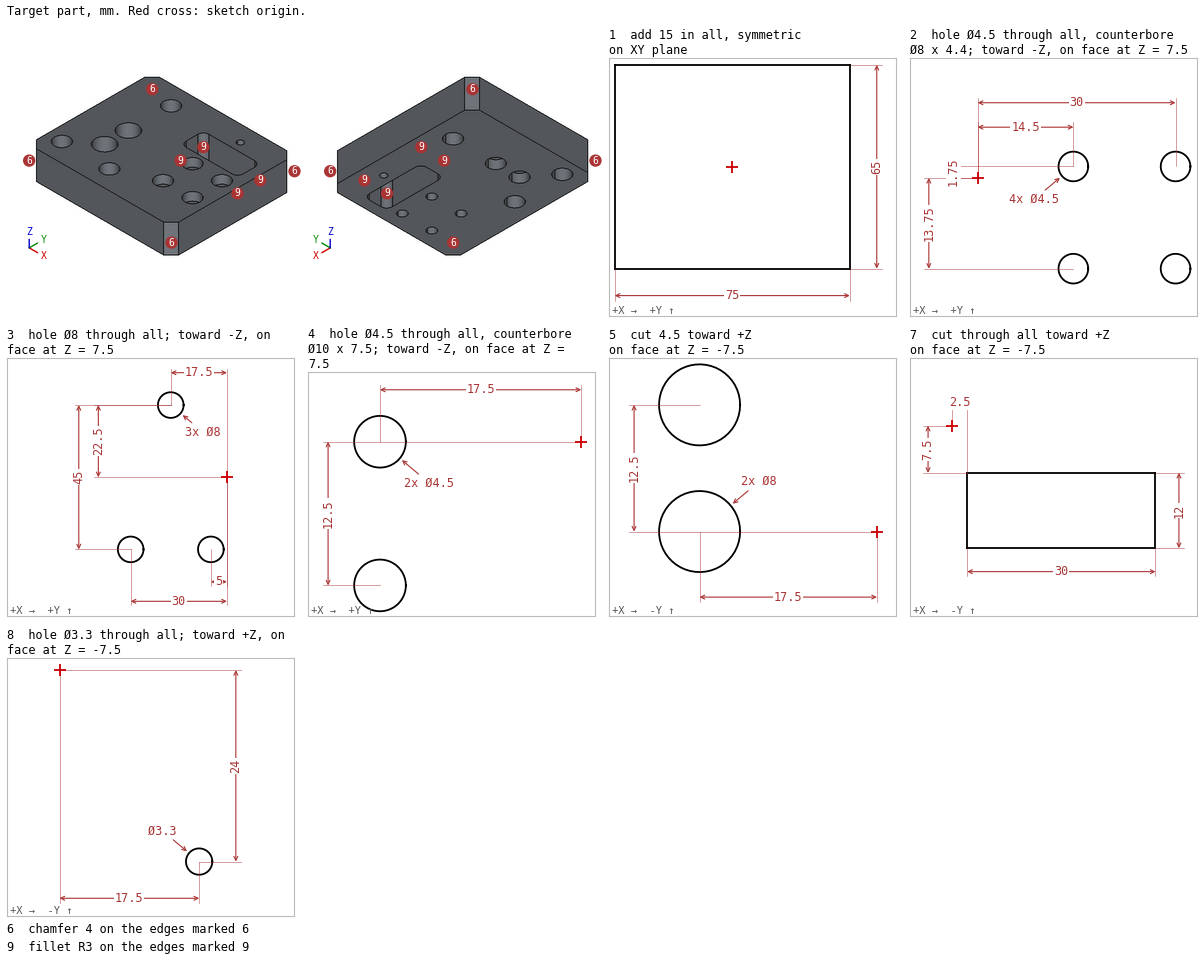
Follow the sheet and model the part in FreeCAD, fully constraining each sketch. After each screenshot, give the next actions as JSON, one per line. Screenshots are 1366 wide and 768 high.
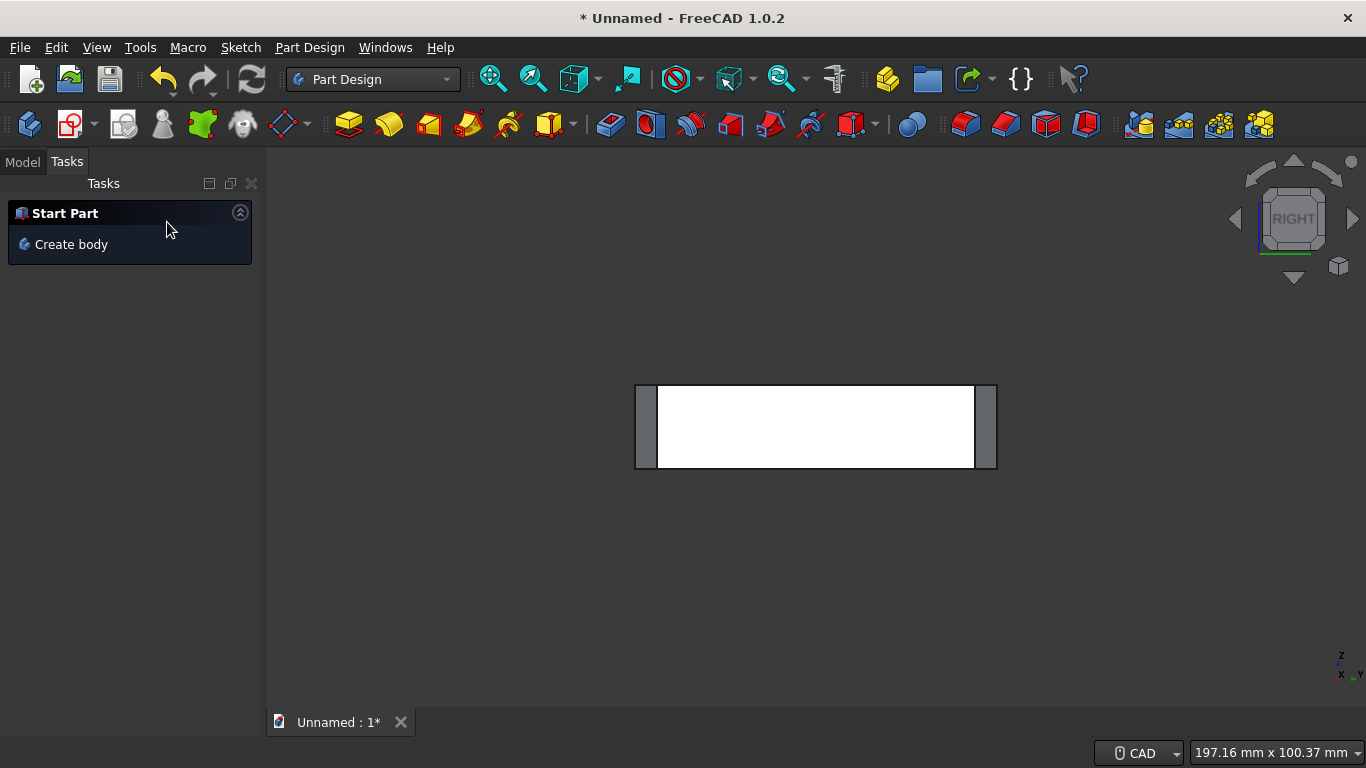
{"action": "key", "text": "v f"}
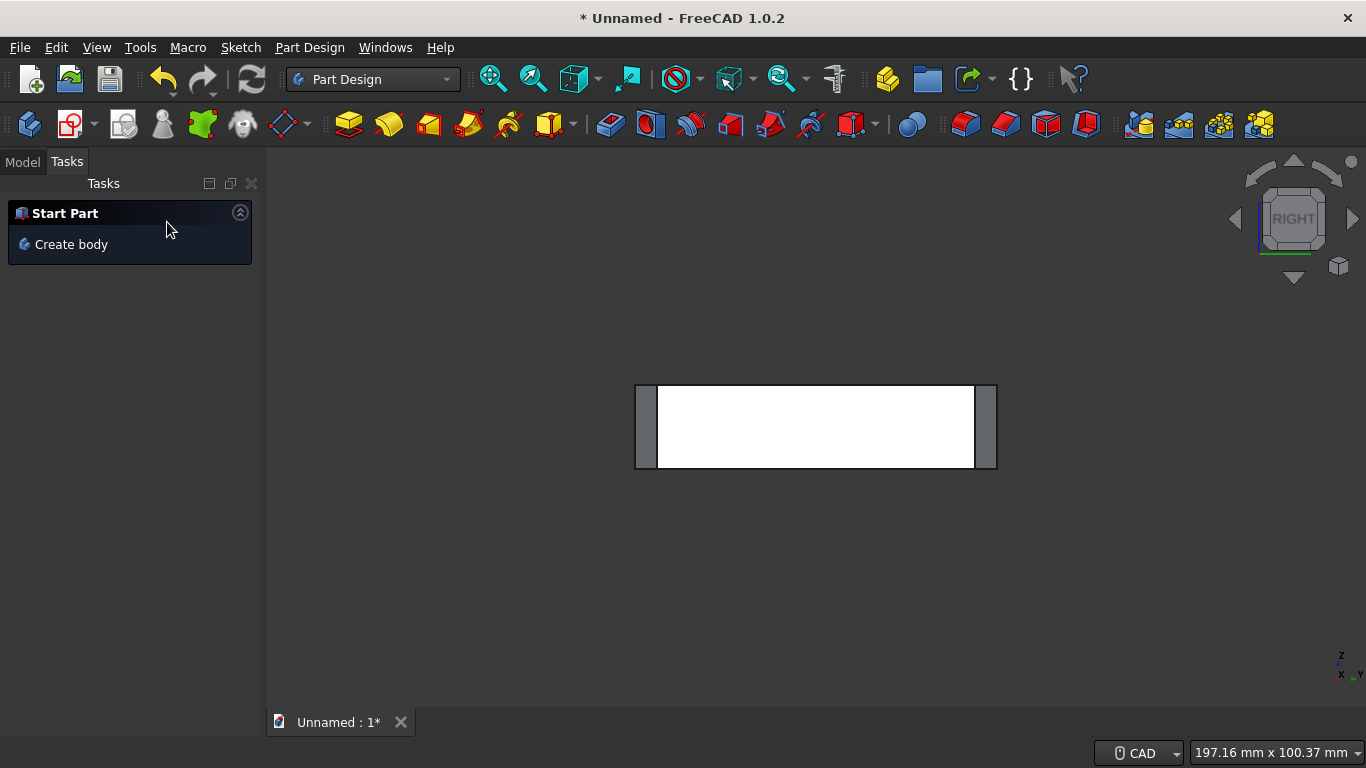
{"action": "key", "text": "5"}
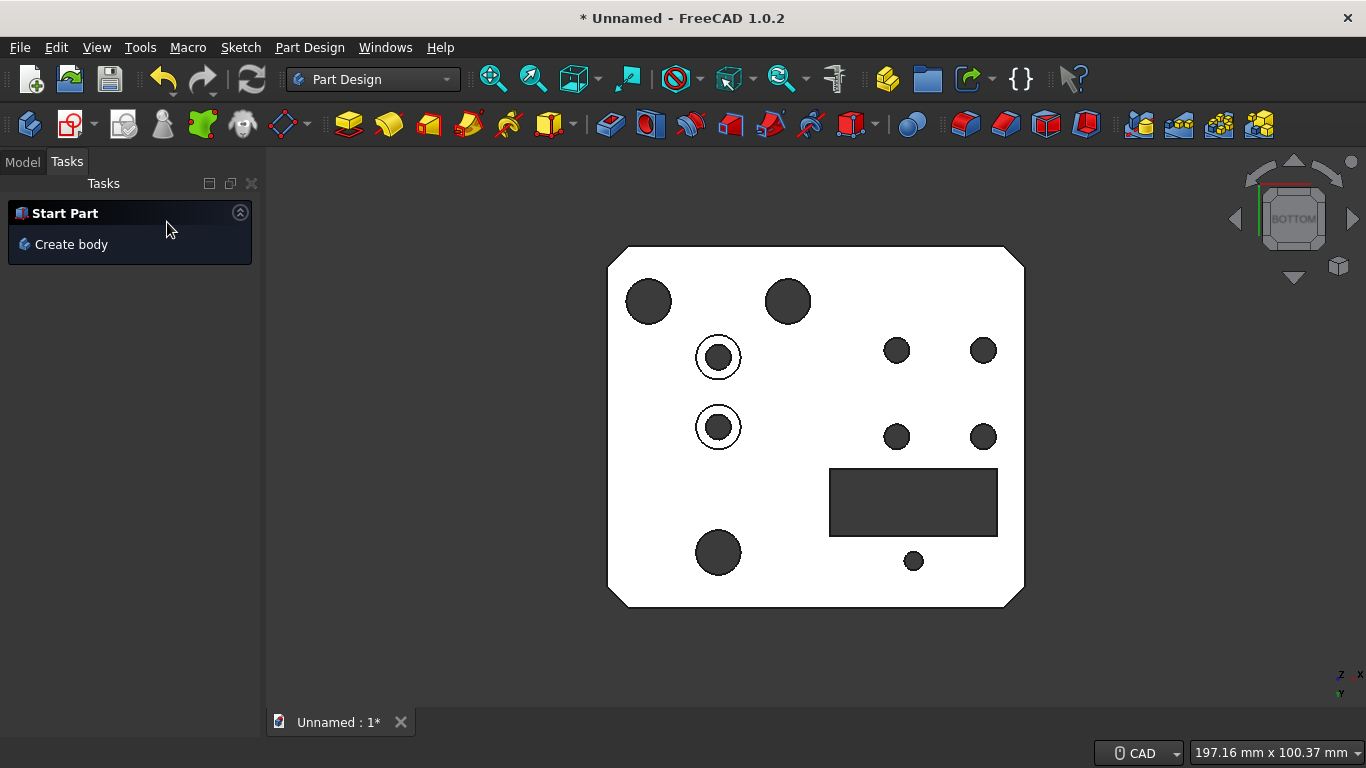
{"action": "key", "text": "4"}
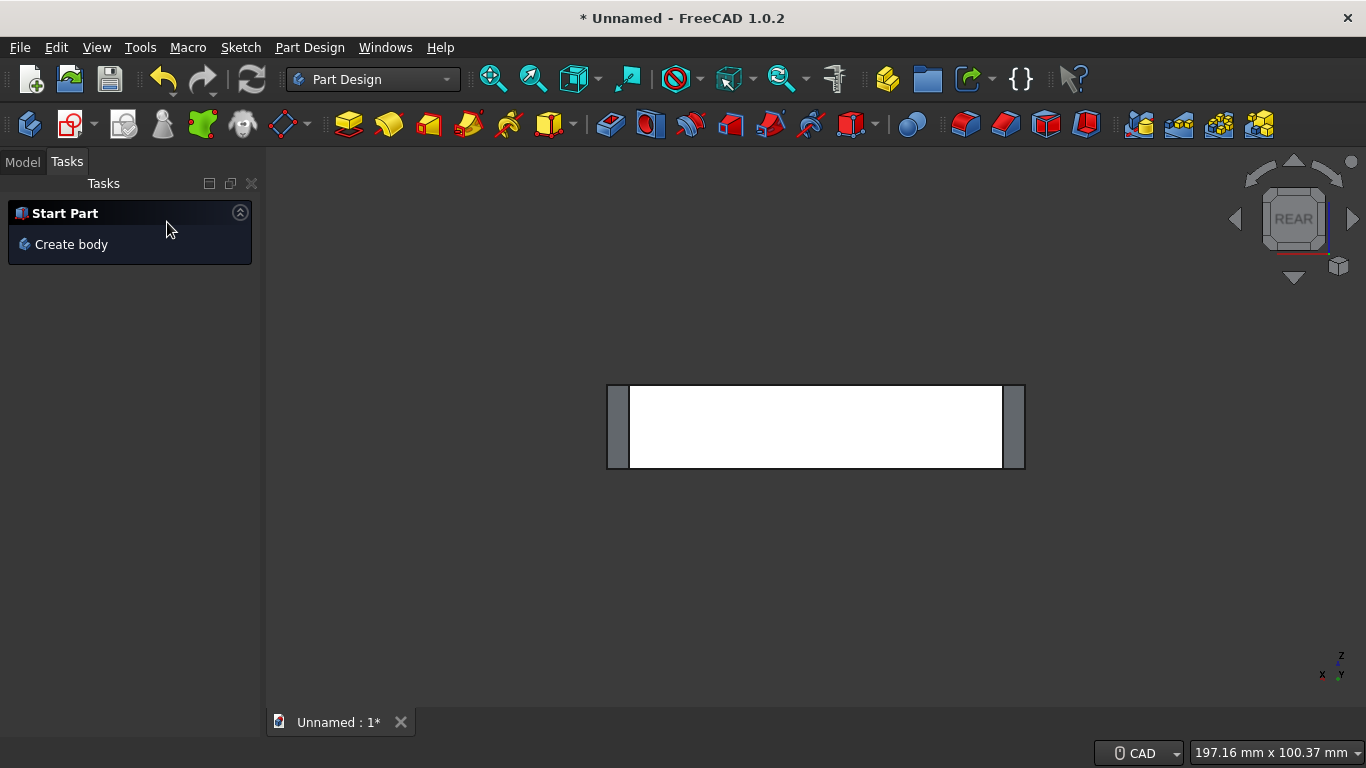
{"action": "left_click", "coordinate": [494, 80]}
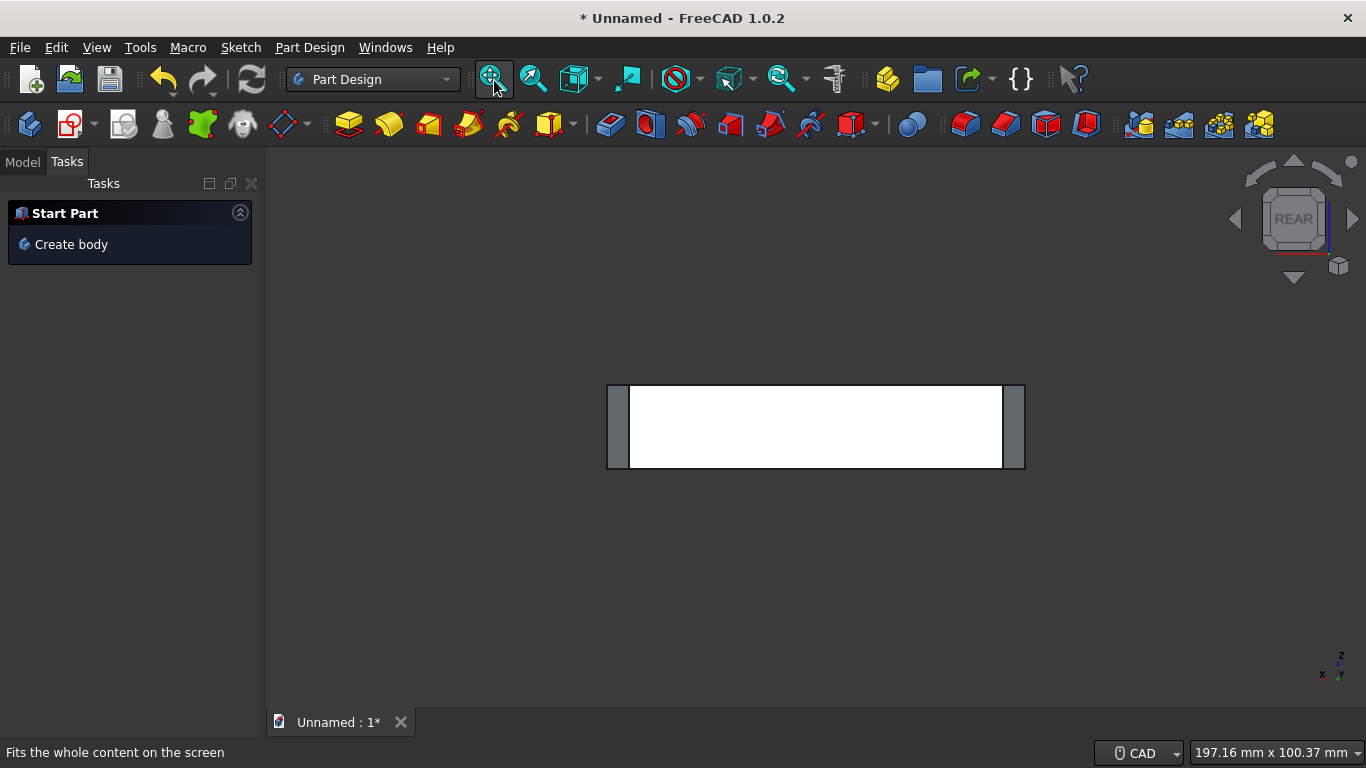
{"action": "key", "text": "6"}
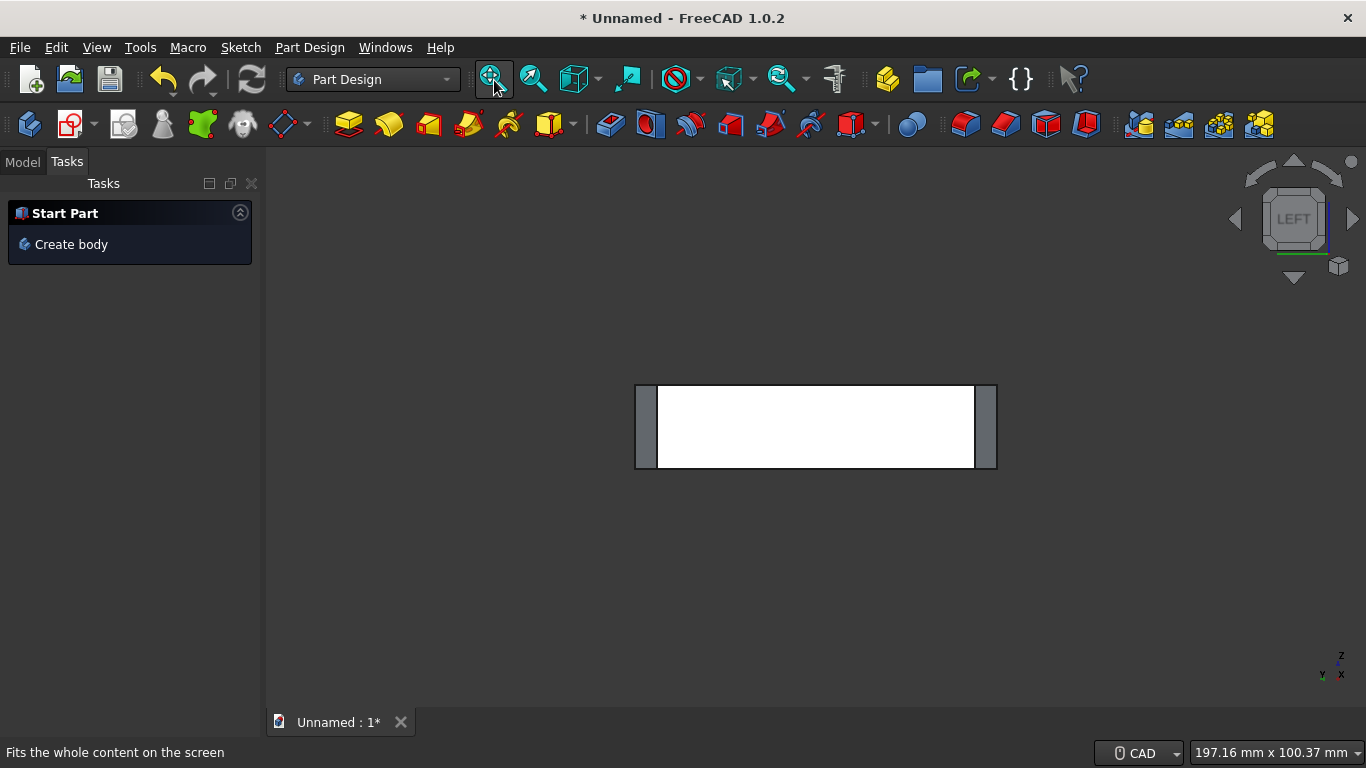
{"action": "key", "text": "v f"}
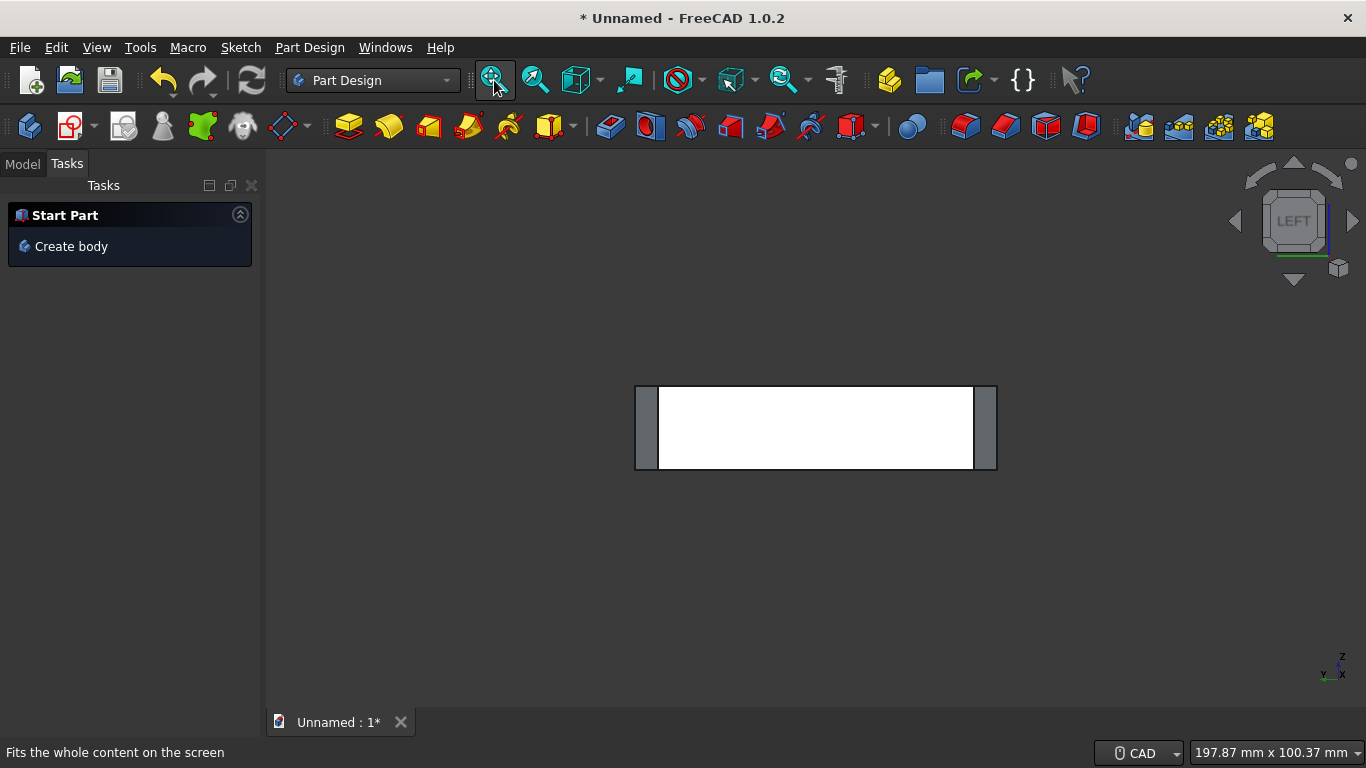
{"action": "key", "text": "v 3"}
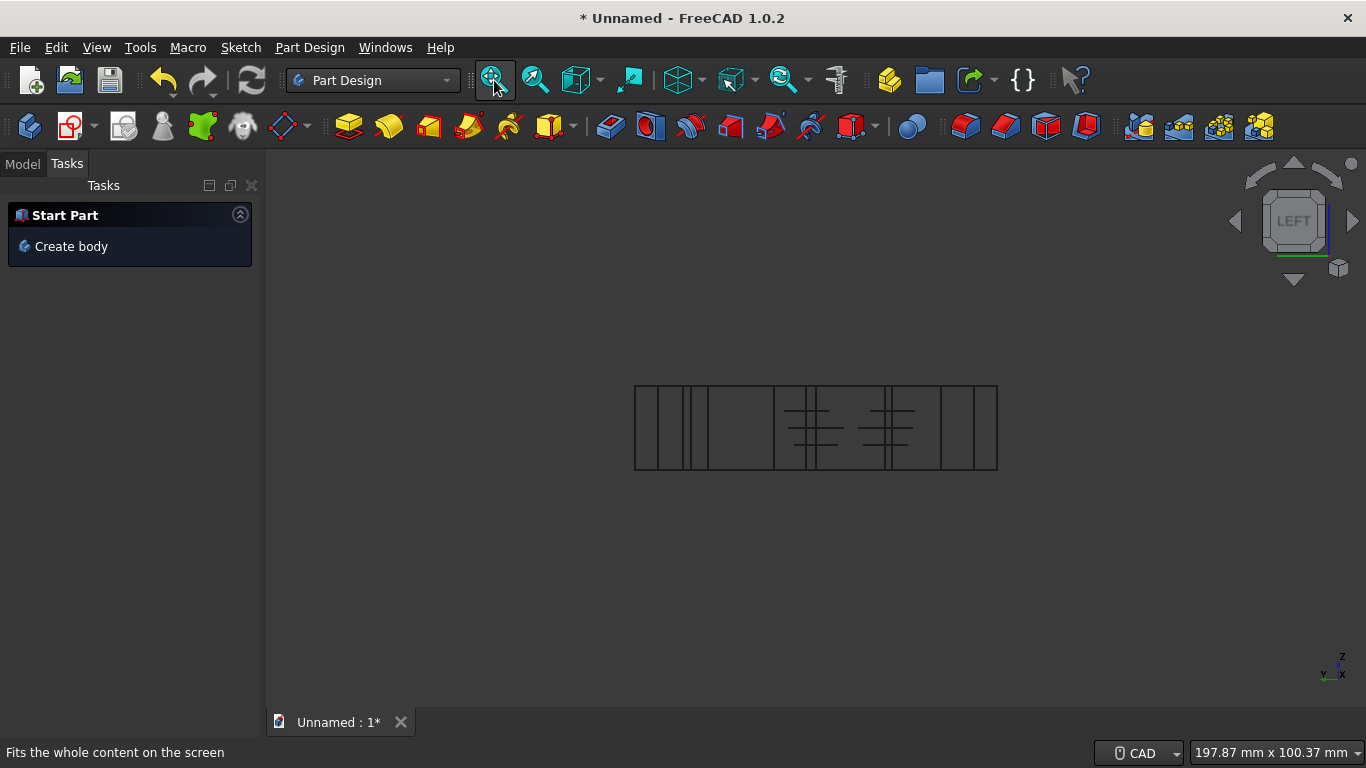
{"action": "key", "text": "0"}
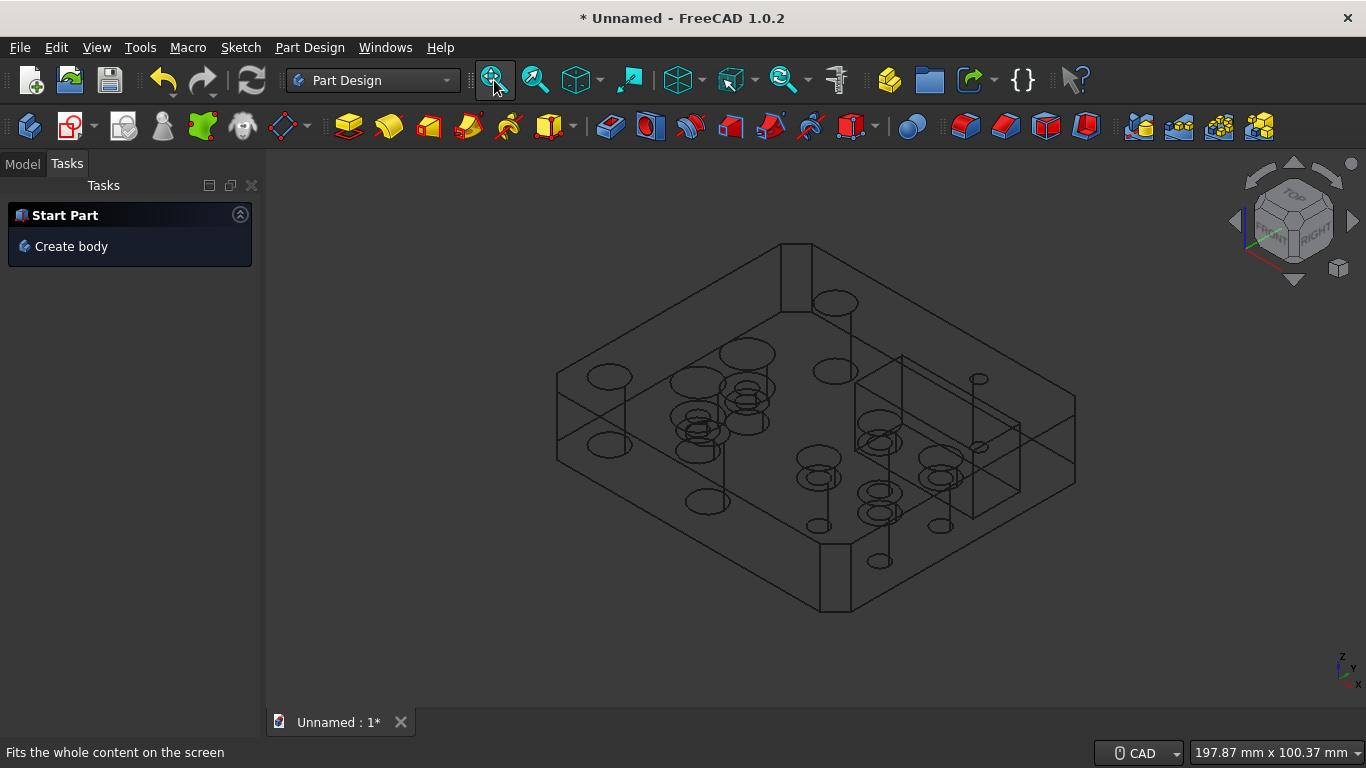
{"action": "left_click", "coordinate": [902, 388]}